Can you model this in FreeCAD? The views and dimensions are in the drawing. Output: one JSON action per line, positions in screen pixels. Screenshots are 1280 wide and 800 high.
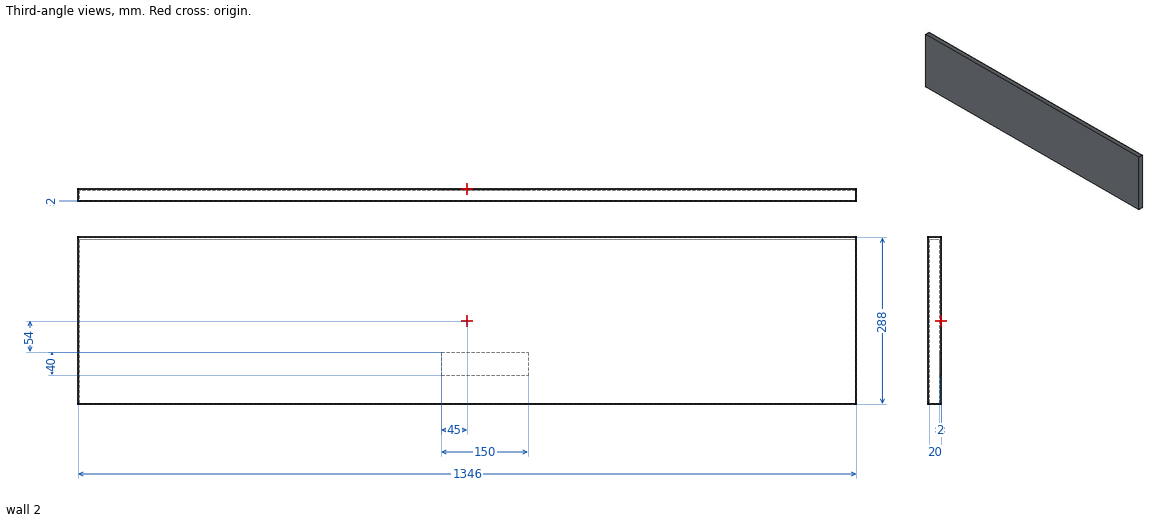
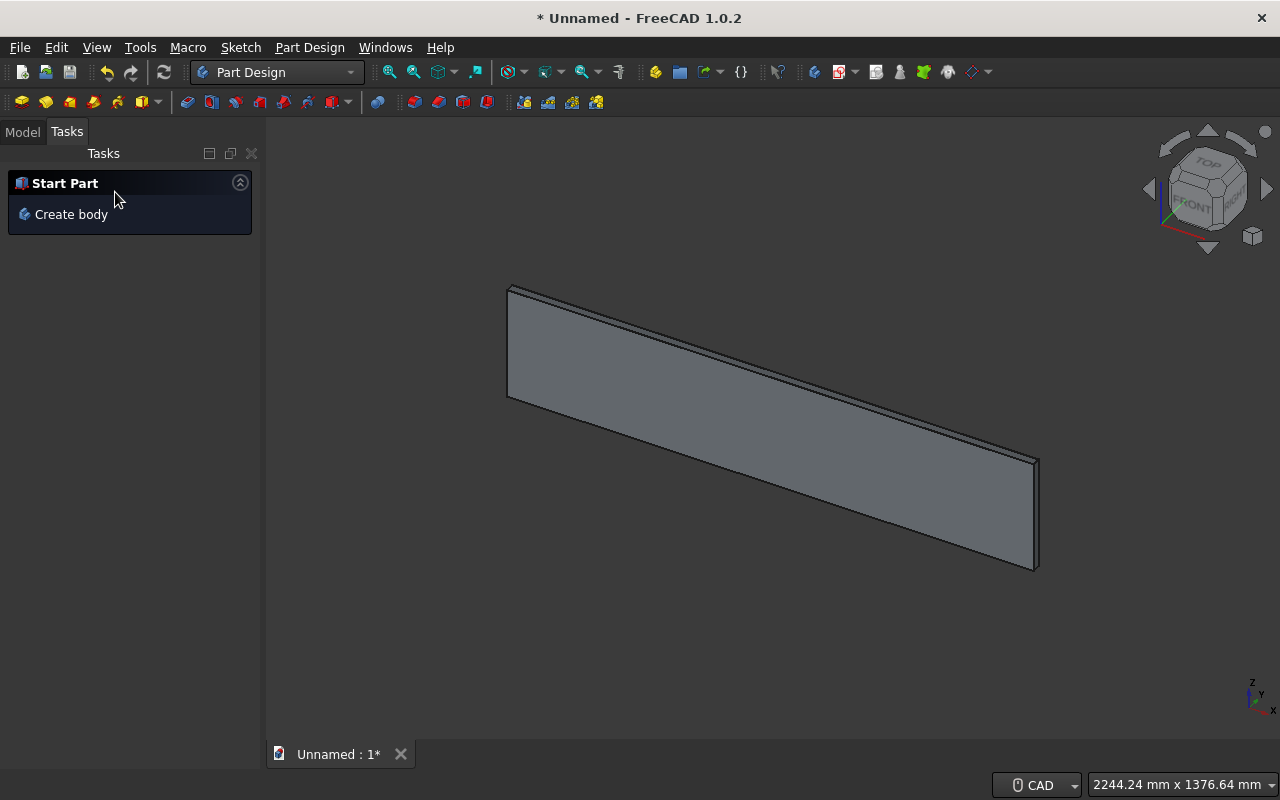
{"action": "key", "text": "0"}